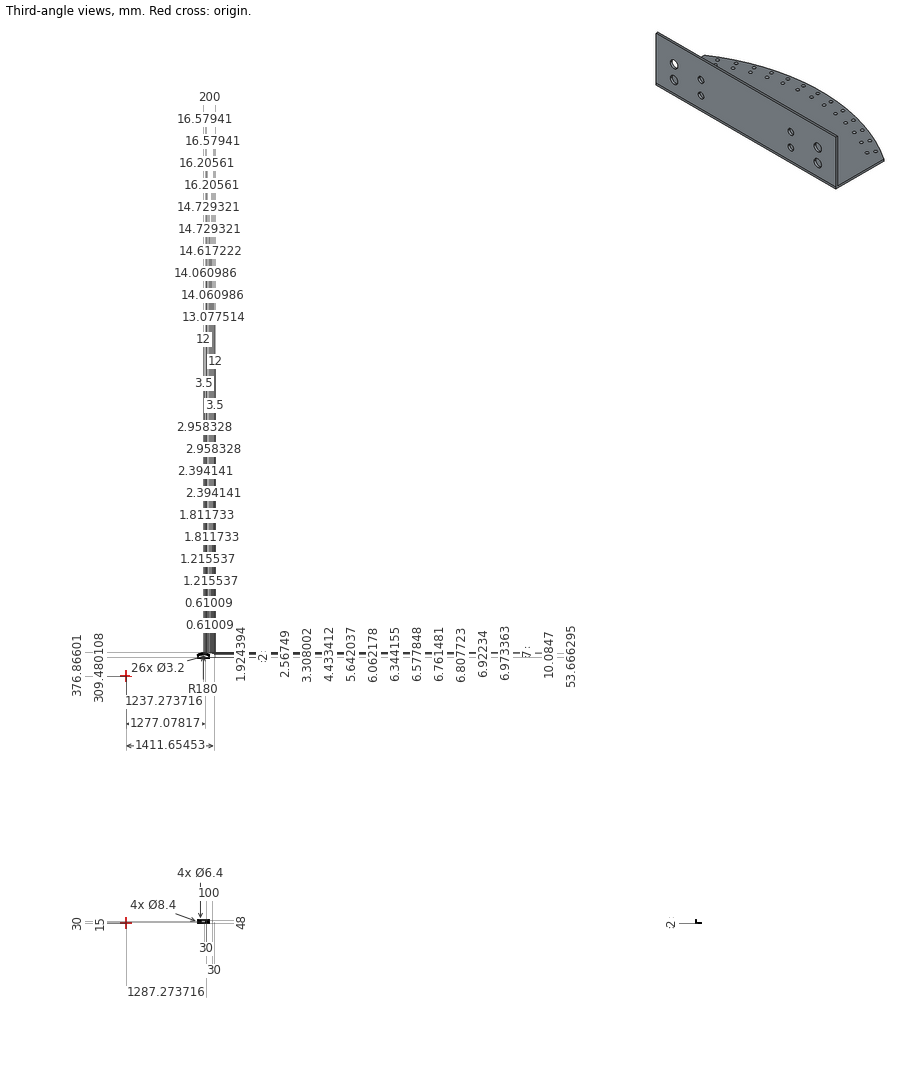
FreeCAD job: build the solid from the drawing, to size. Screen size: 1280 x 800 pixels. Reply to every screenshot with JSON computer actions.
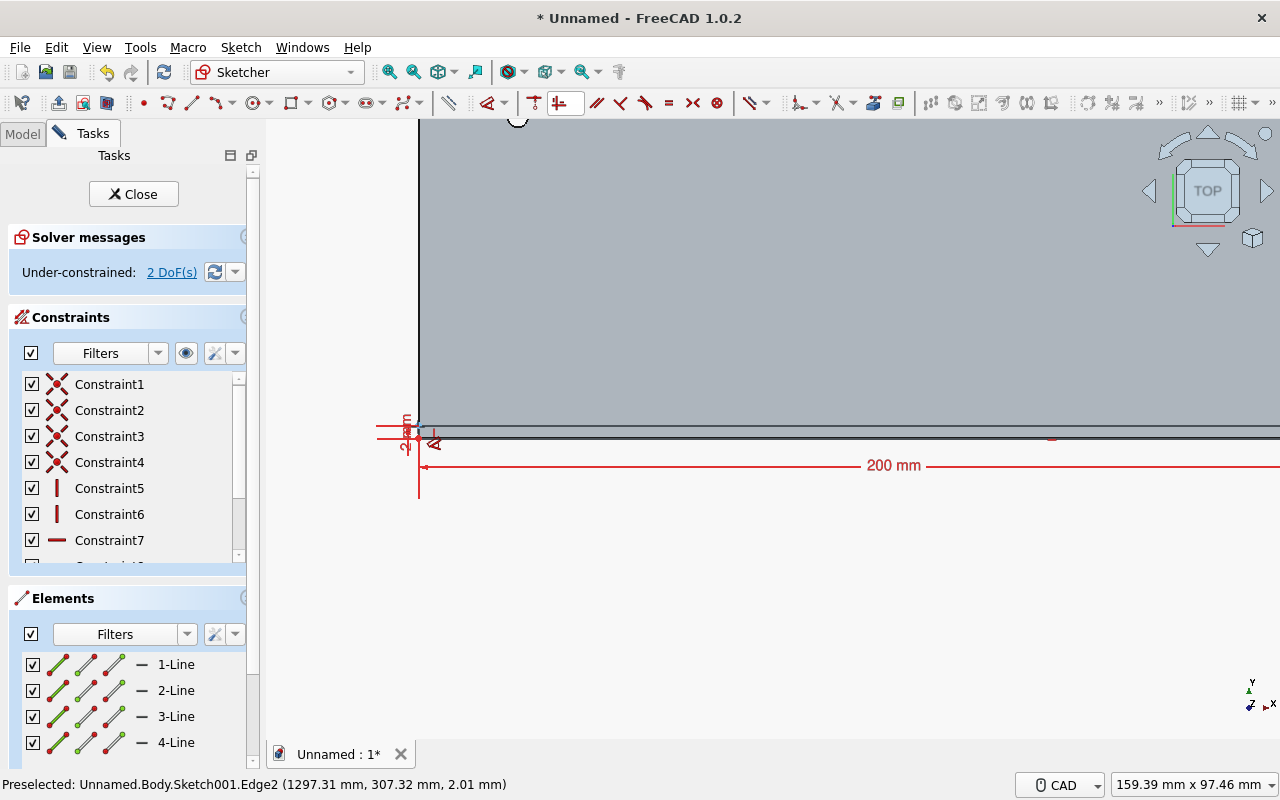
{"action": "left_click", "coordinate": [419, 426]}
{"action": "left_click", "coordinate": [453, 568]}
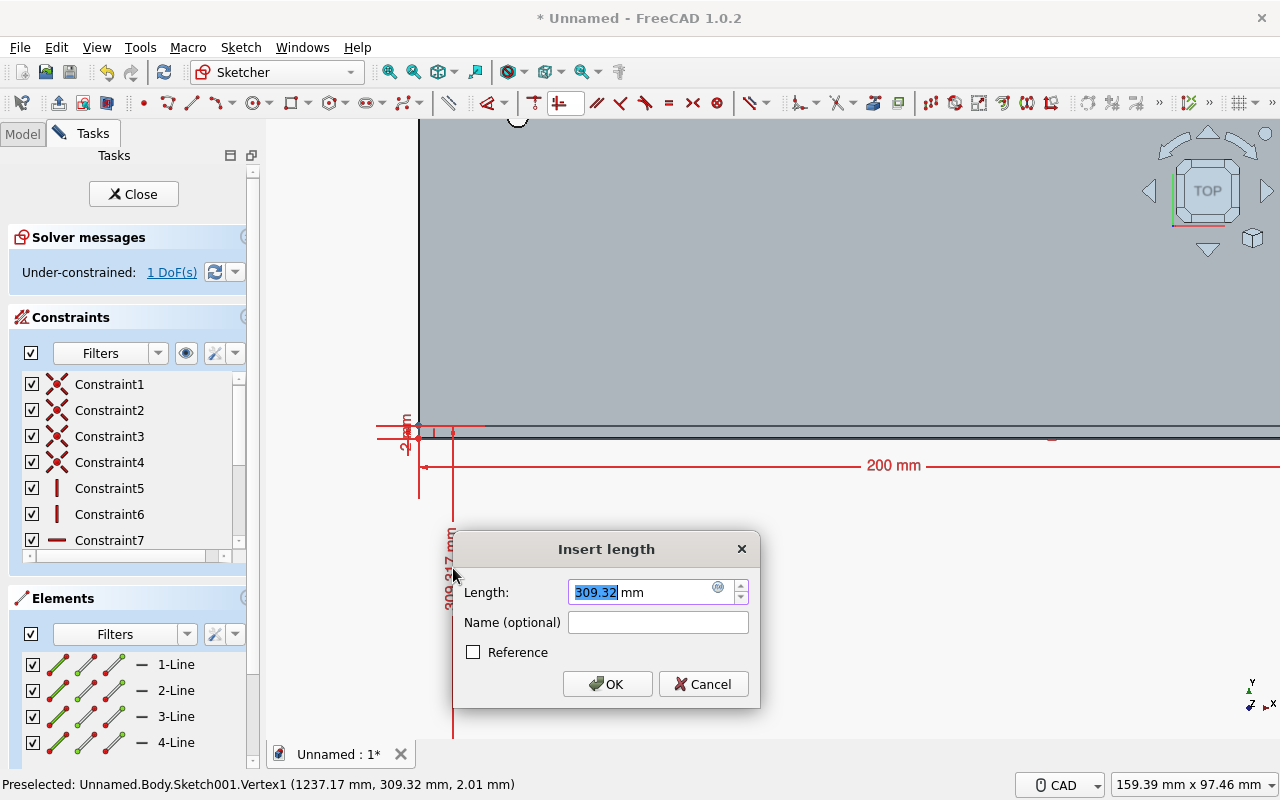
{"action": "type", "text": "309.480108"}
{"action": "key", "text": "Return"}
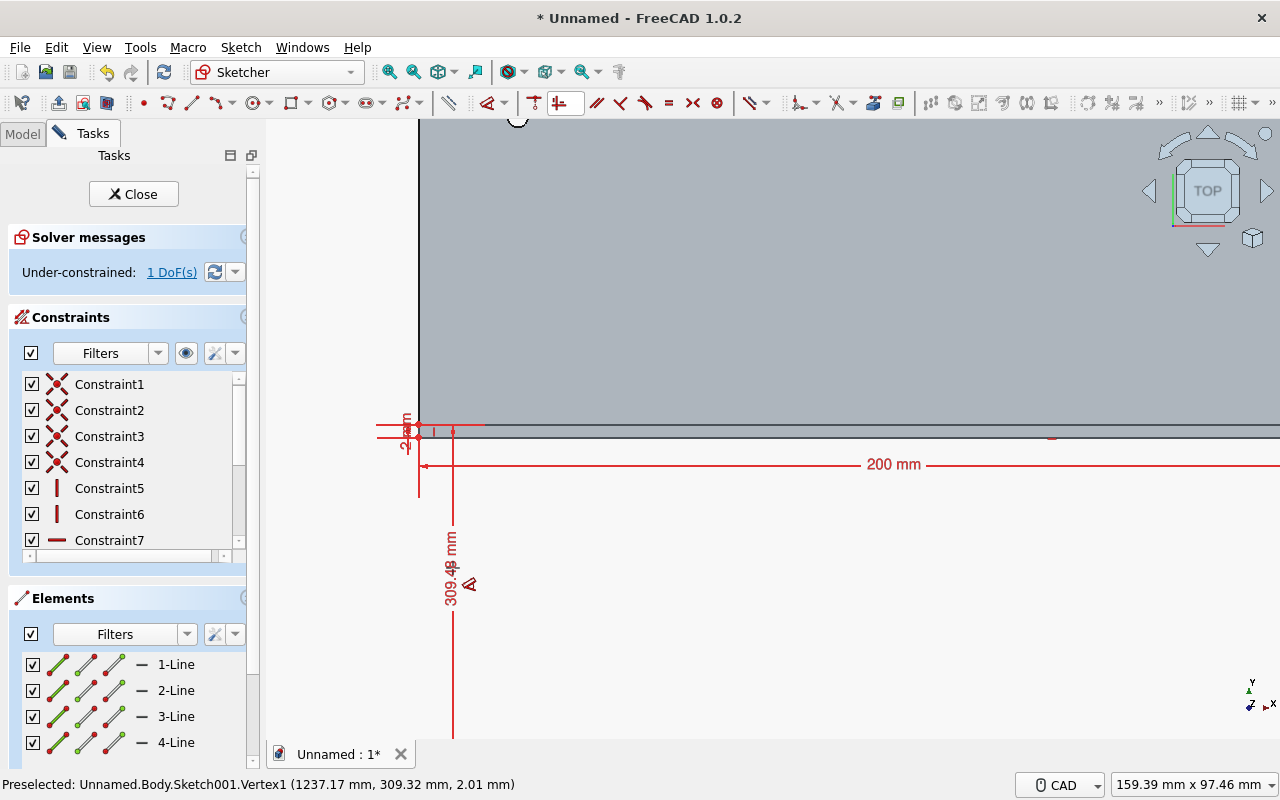
{"action": "left_click", "coordinate": [419, 425]}
{"action": "left_click", "coordinate": [356, 391]}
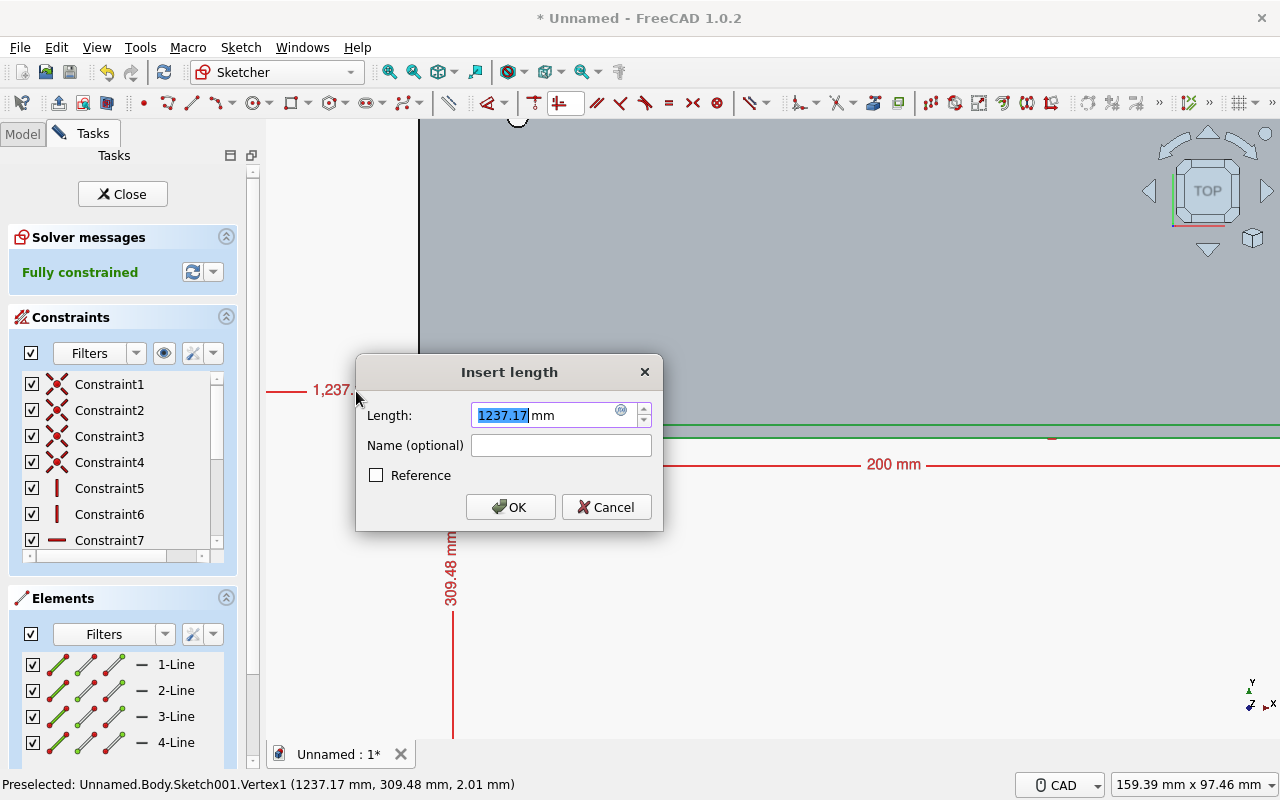
{"action": "type", "text": "1237.273716"}
{"action": "key", "text": "Return"}
{"action": "key", "text": "Escape"}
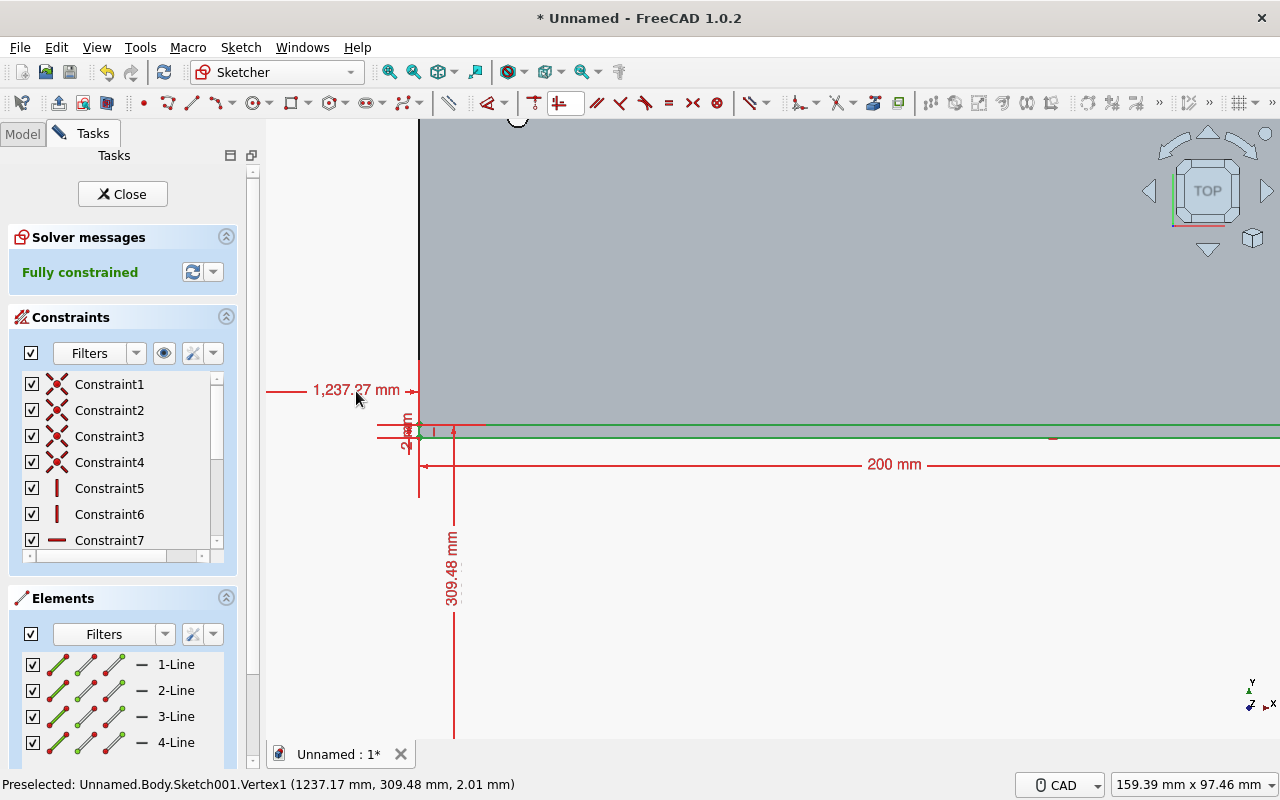
{"action": "left_click", "coordinate": [123, 194]}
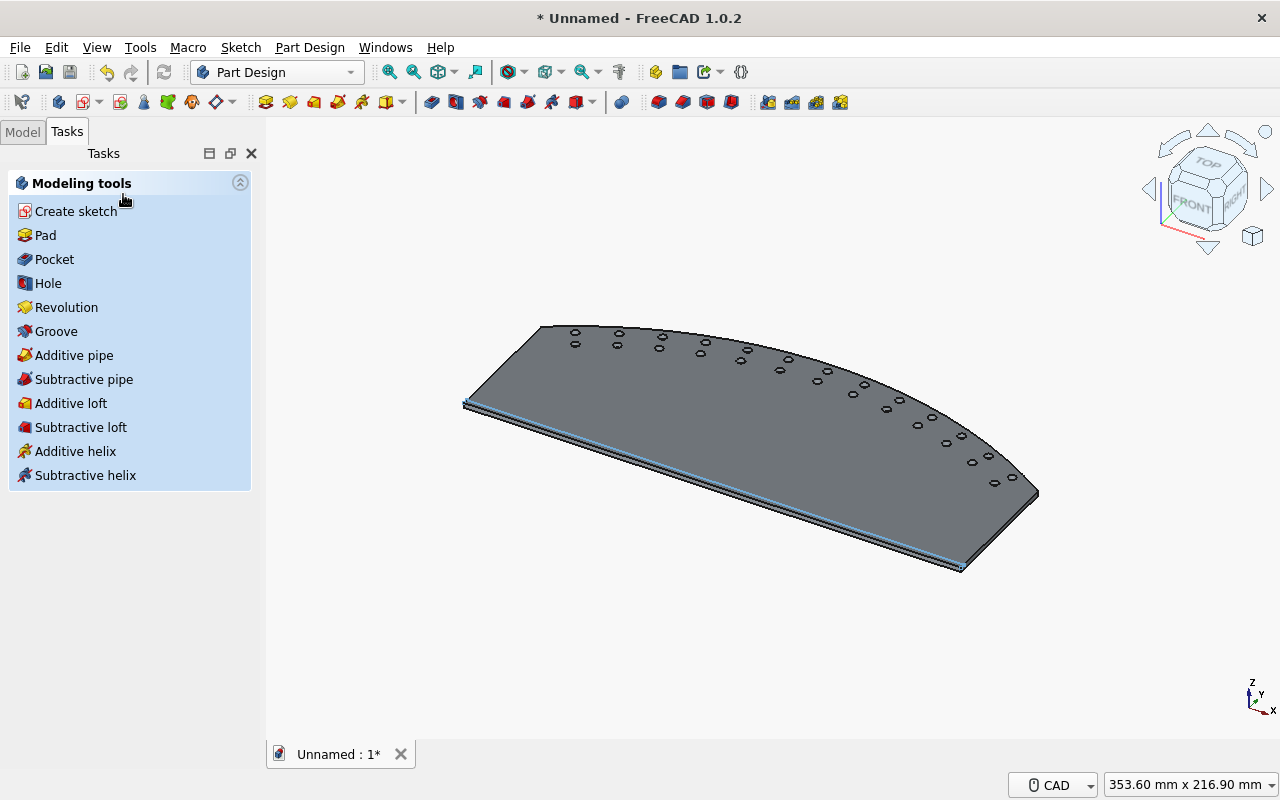
{"action": "left_click", "coordinate": [266, 102]}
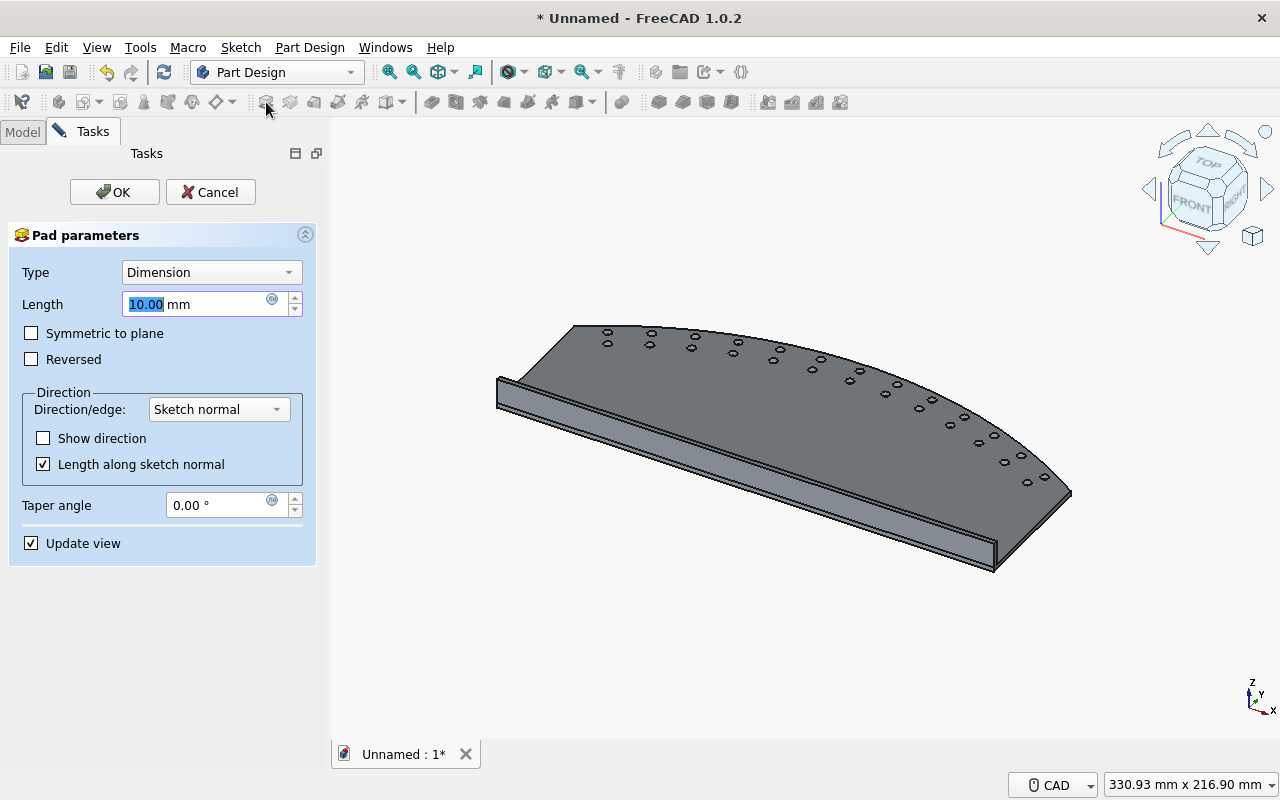
{"action": "type", "text": "48"}
{"action": "key", "text": "Tab"}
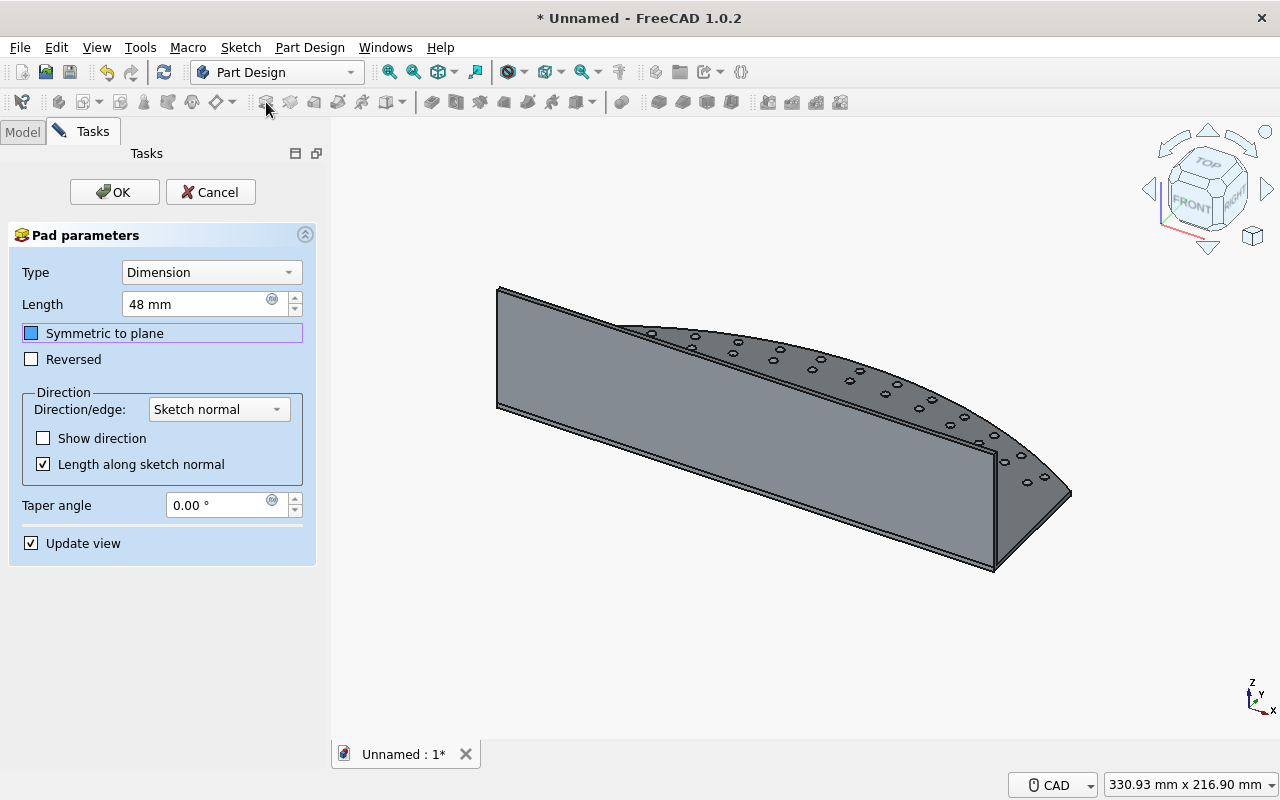
{"action": "left_click", "coordinate": [115, 192]}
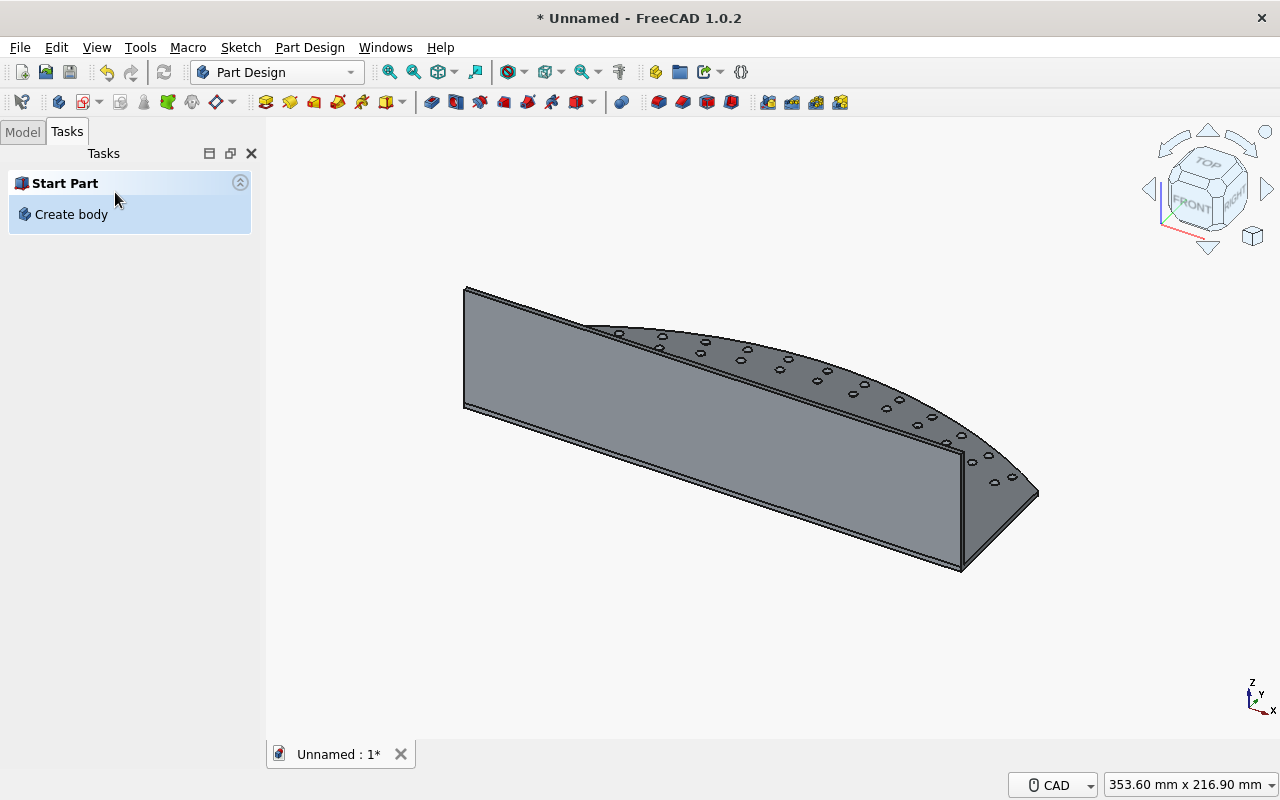
{"action": "key", "text": "4"}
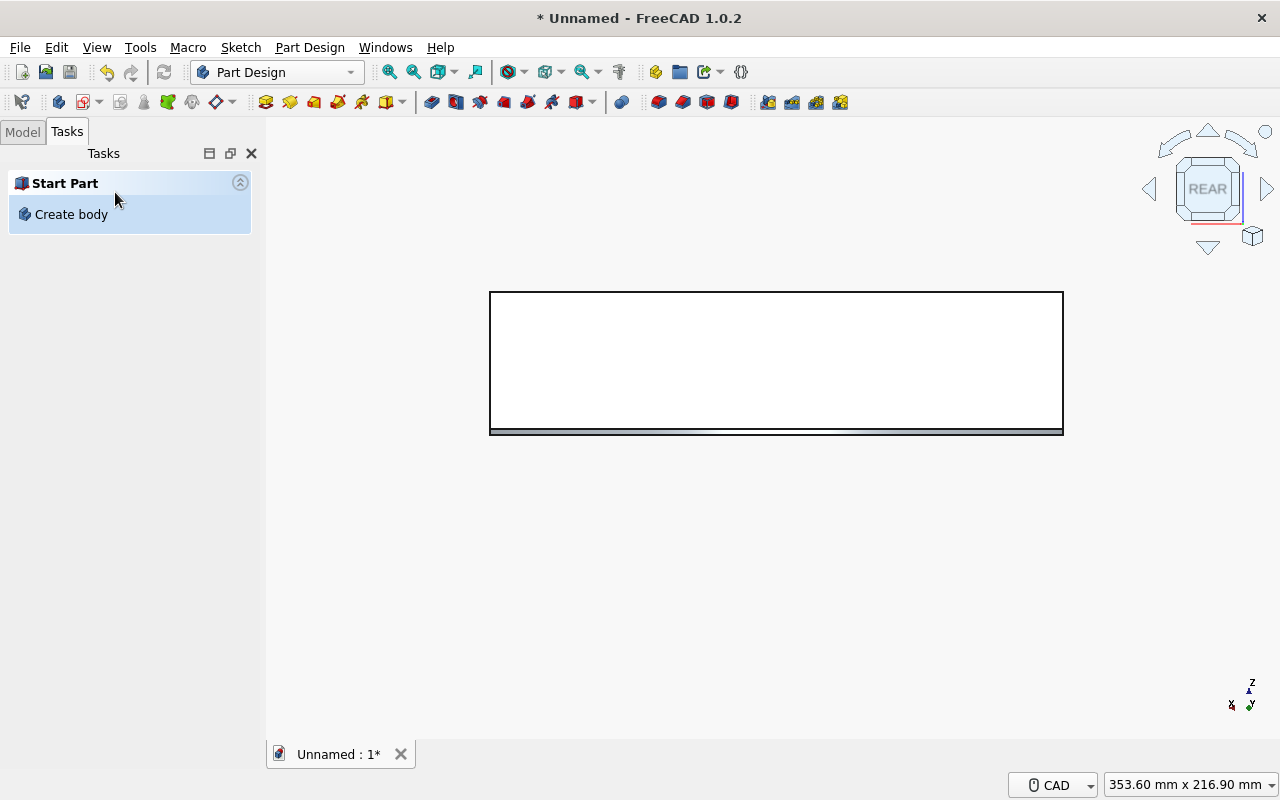
{"action": "left_click", "coordinate": [612, 360]}